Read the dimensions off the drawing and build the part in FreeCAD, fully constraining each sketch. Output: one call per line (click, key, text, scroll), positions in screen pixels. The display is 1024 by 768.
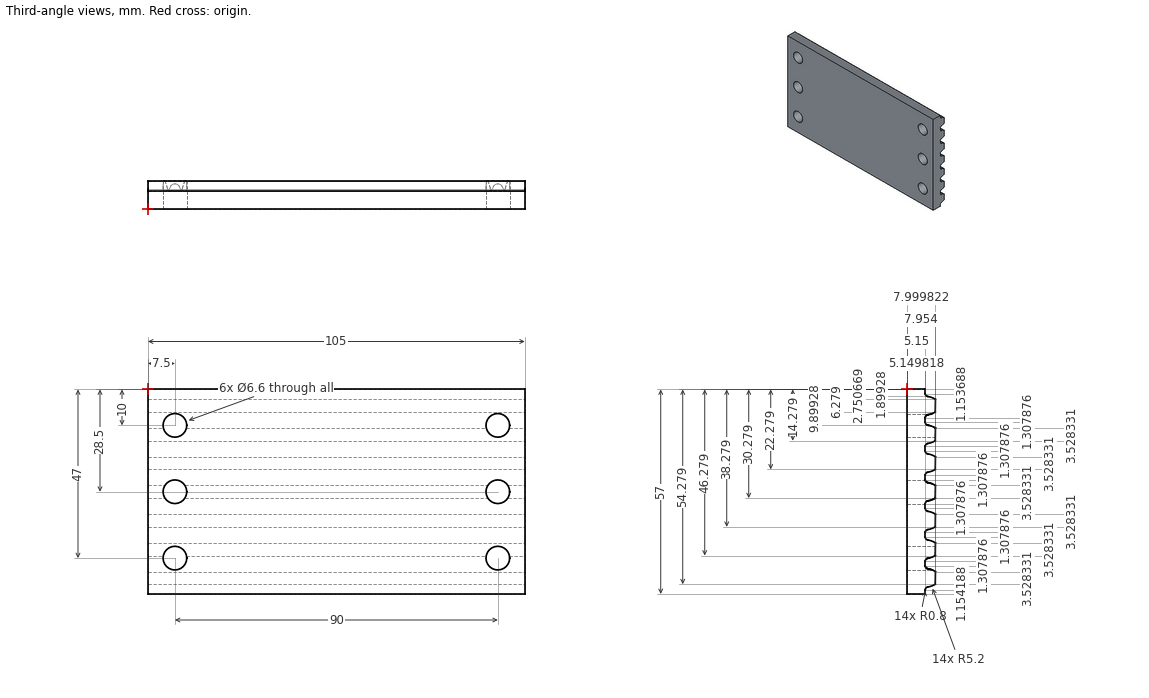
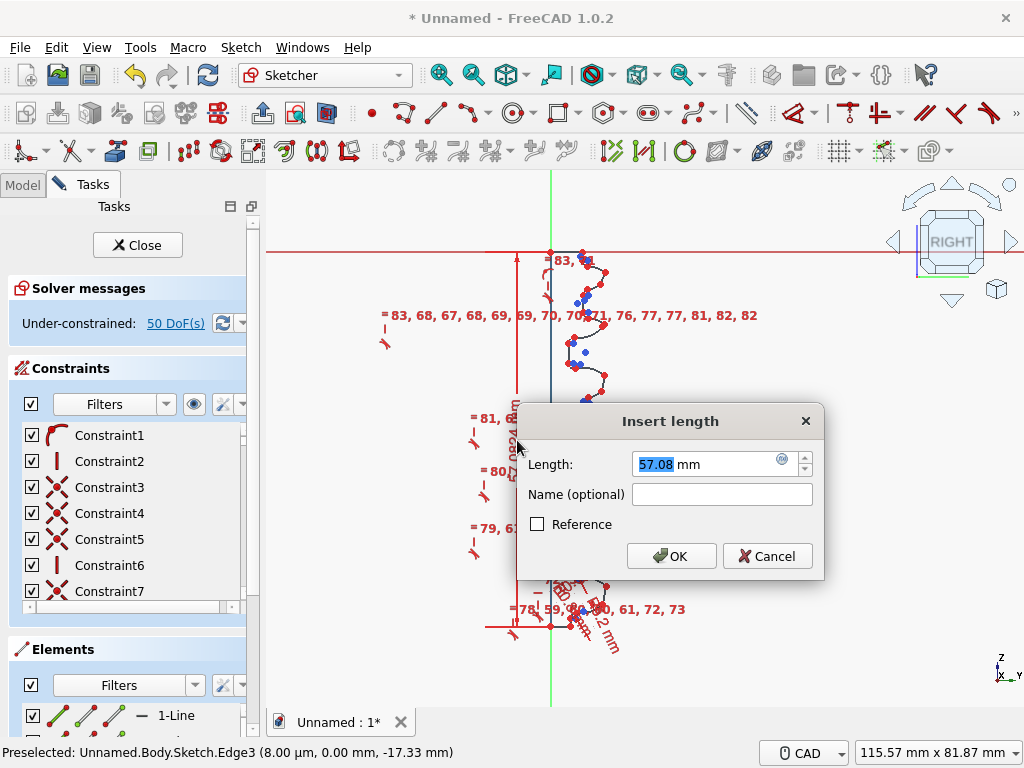
text(57)
key(Return)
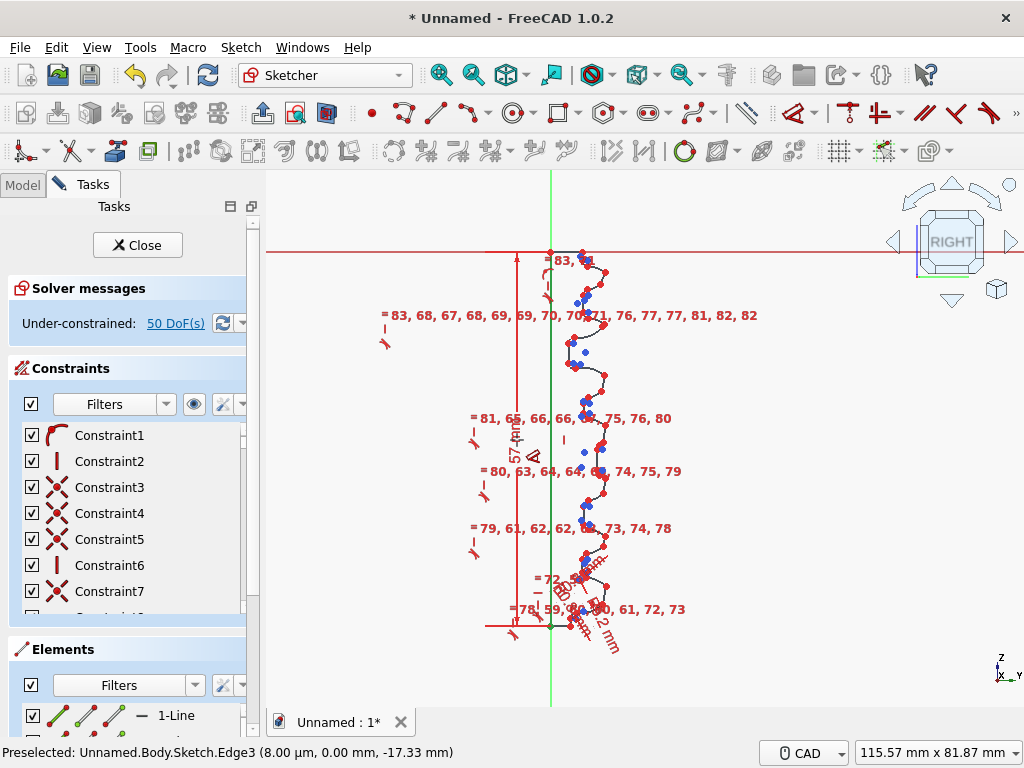
scroll(573, 252, up, 2)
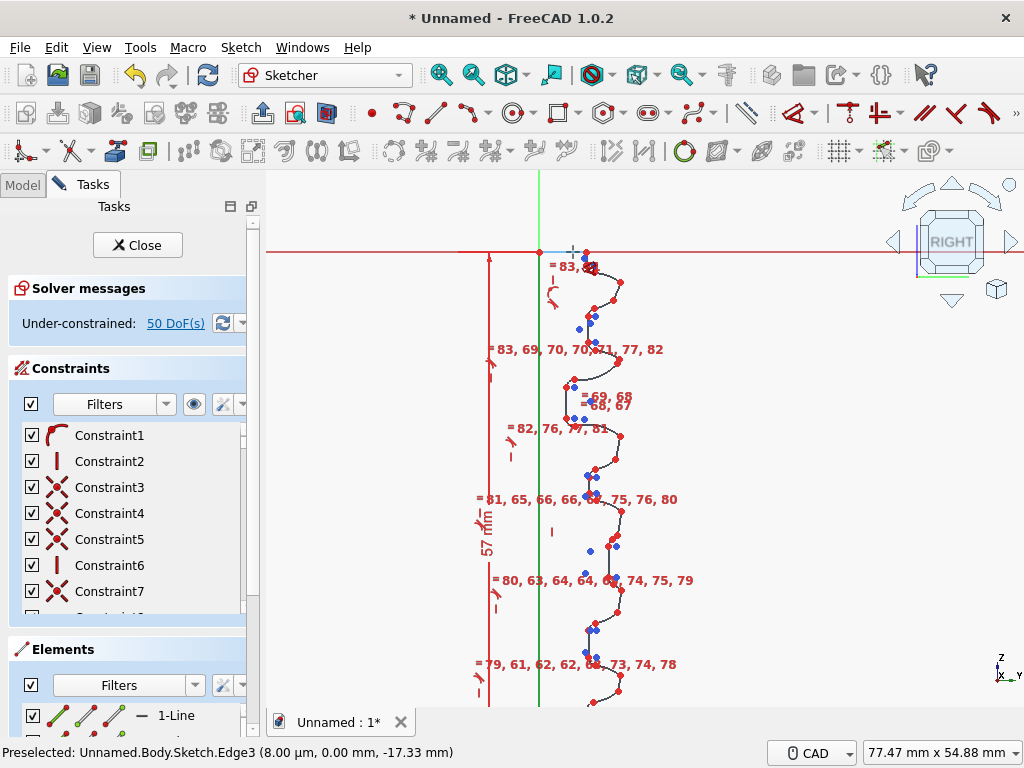
click(573, 252)
click(563, 218)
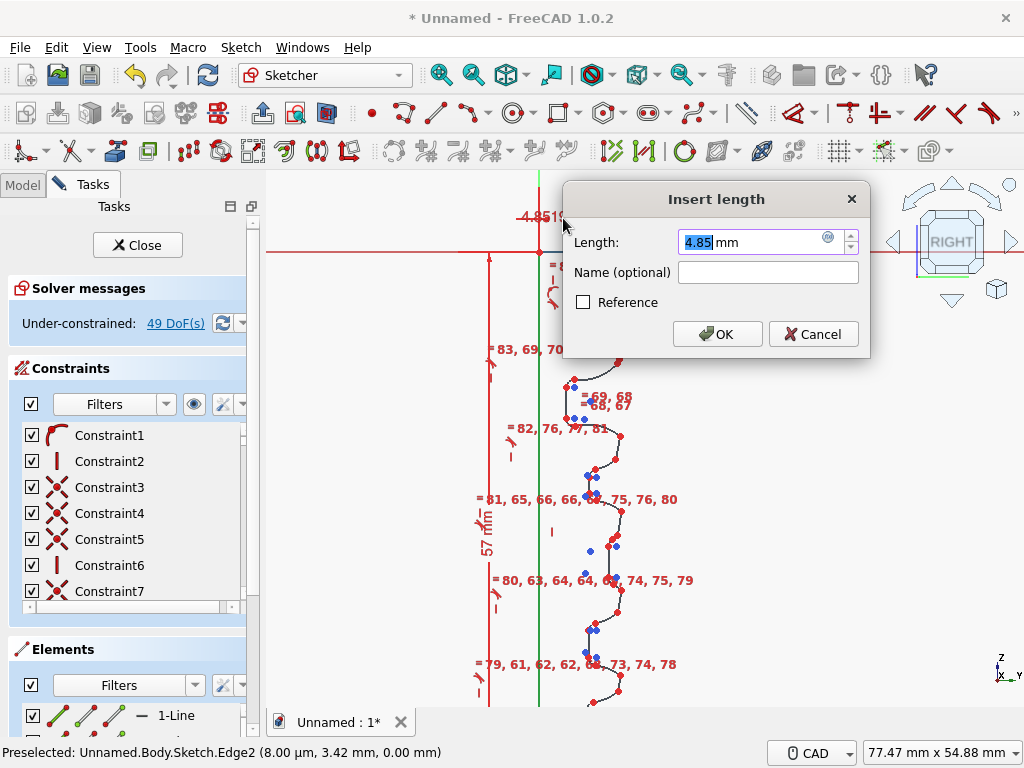
text(5.15)
key(Return)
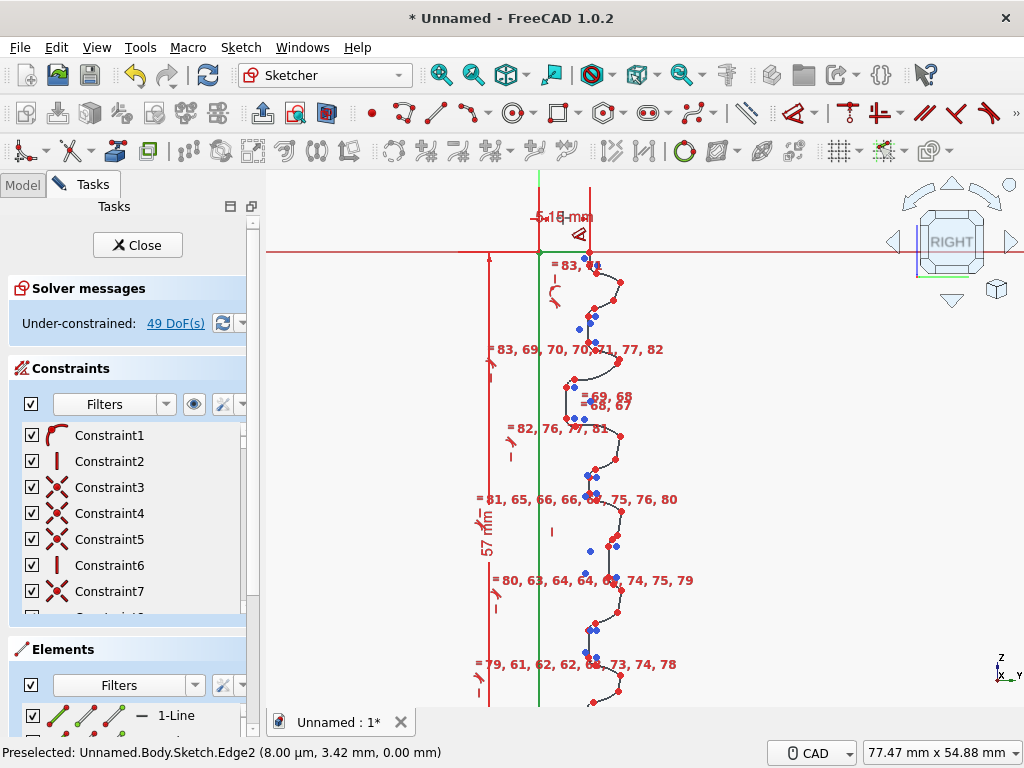
scroll(572, 250, down, 2)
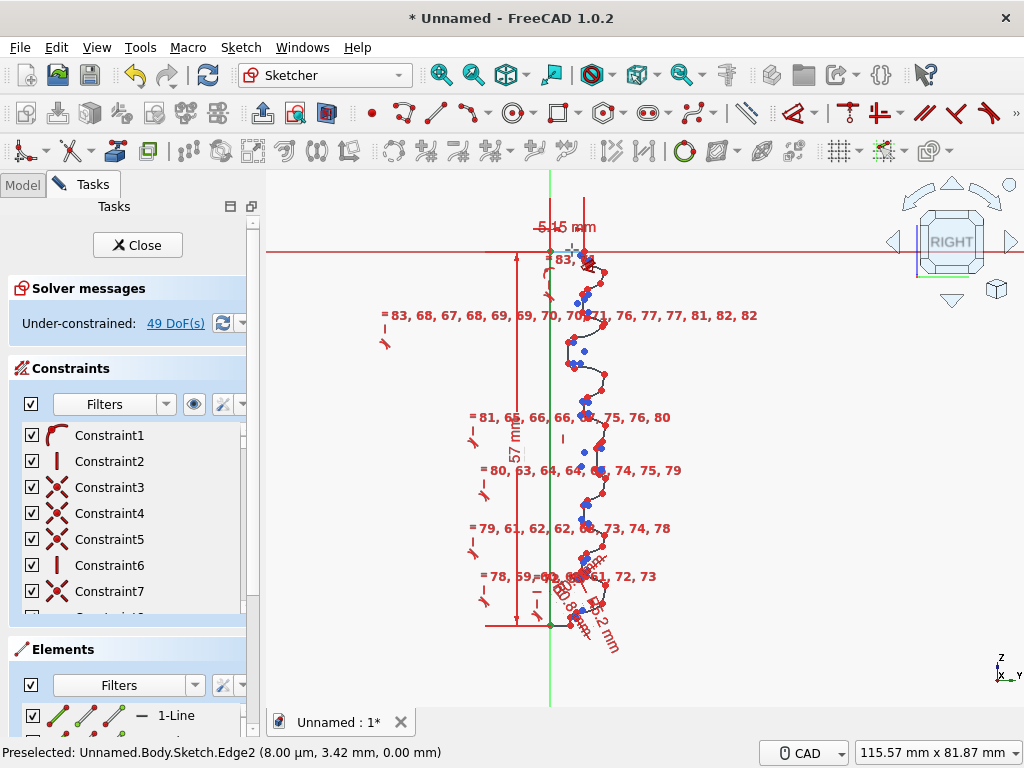
scroll(558, 626, up, 3)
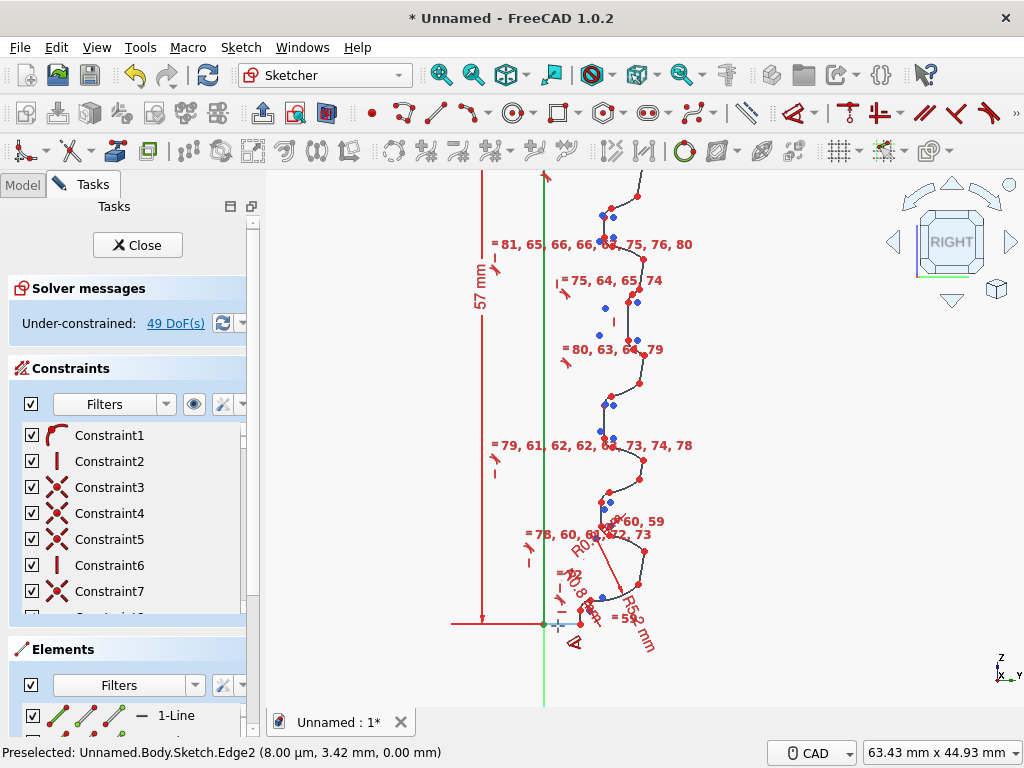
click(558, 624)
click(562, 658)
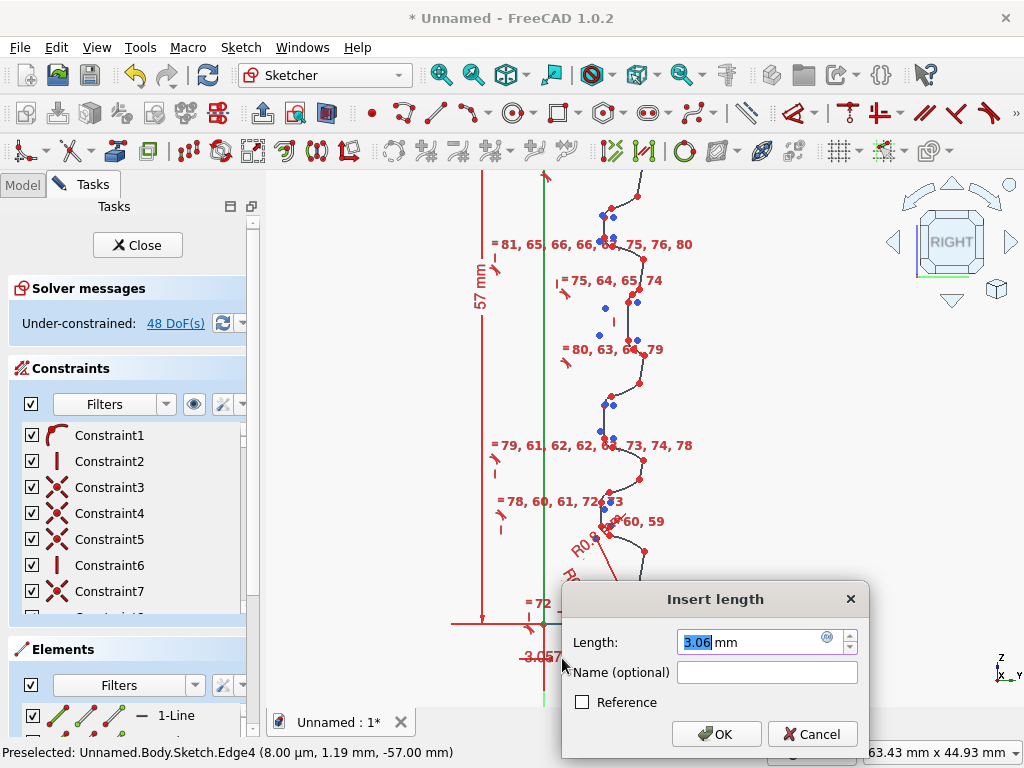
text(5.15)
key(Return)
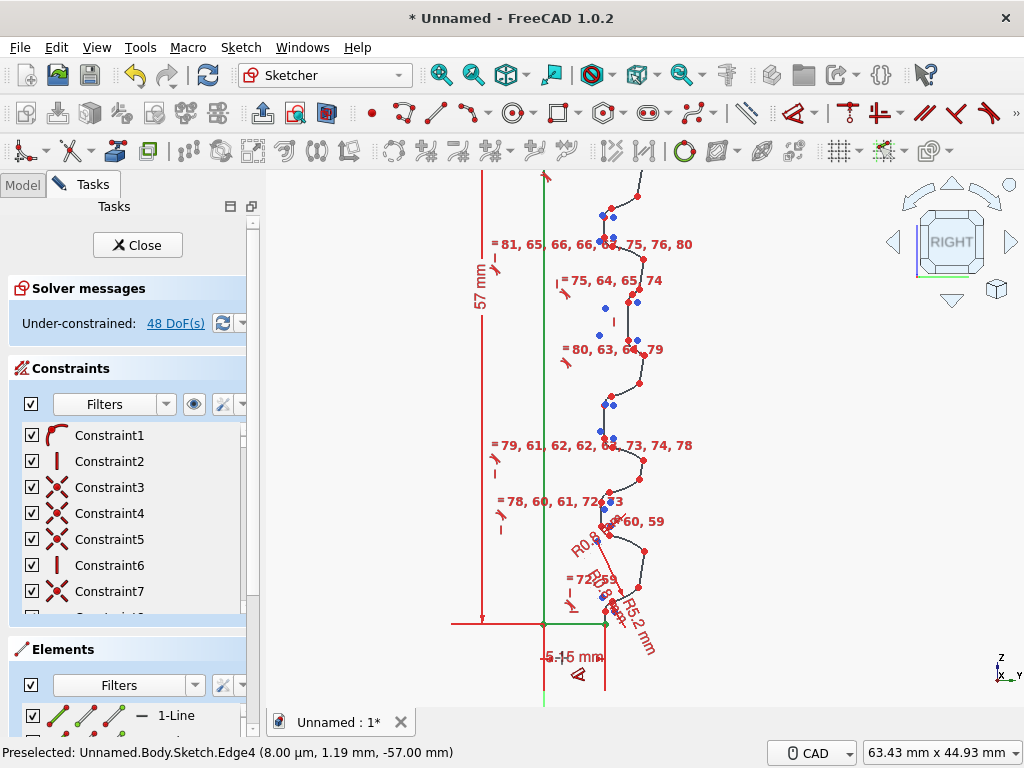
scroll(601, 526, up, 2)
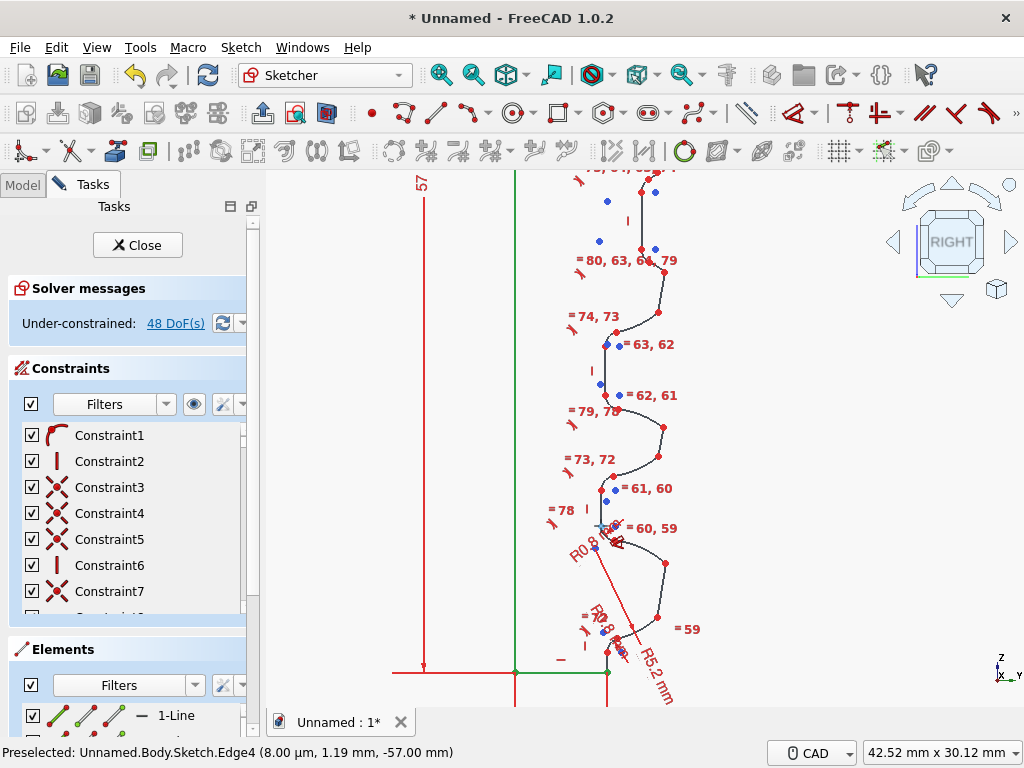
click(601, 526)
click(558, 584)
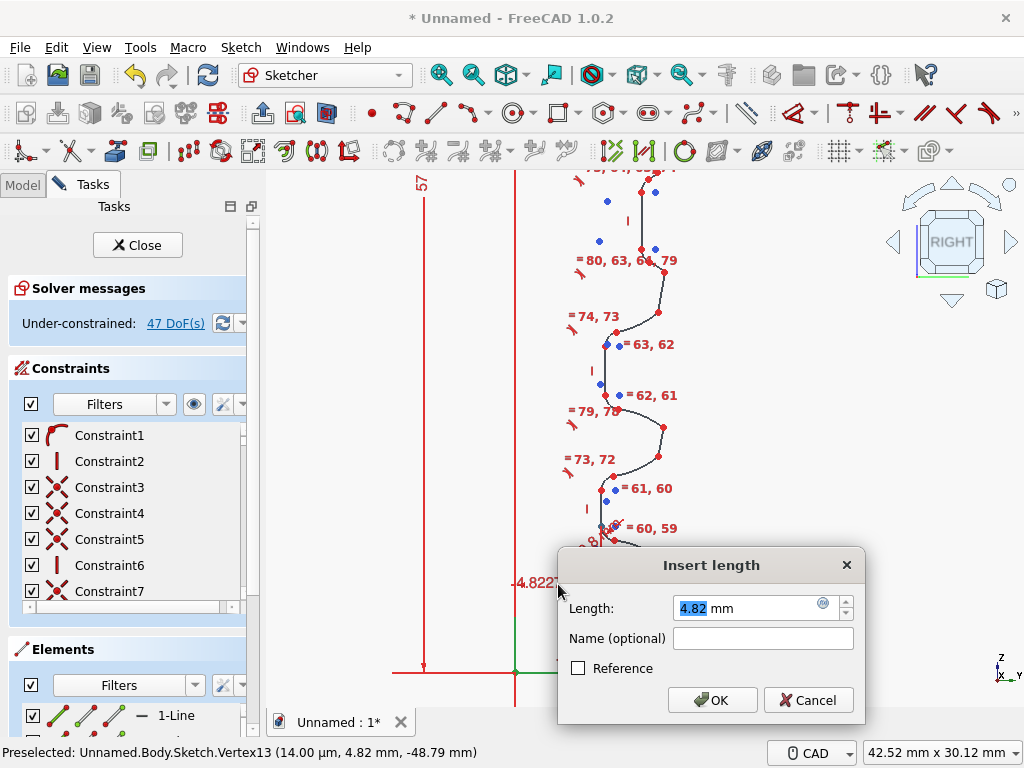
text(5.15)
key(Return)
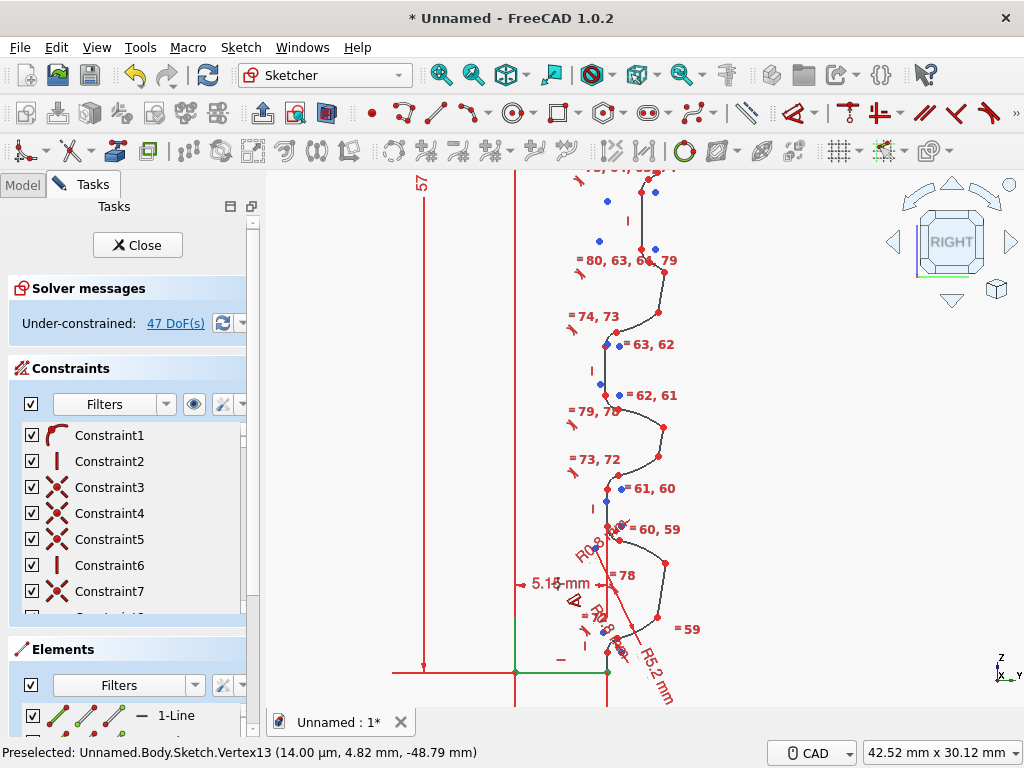
click(605, 395)
click(560, 429)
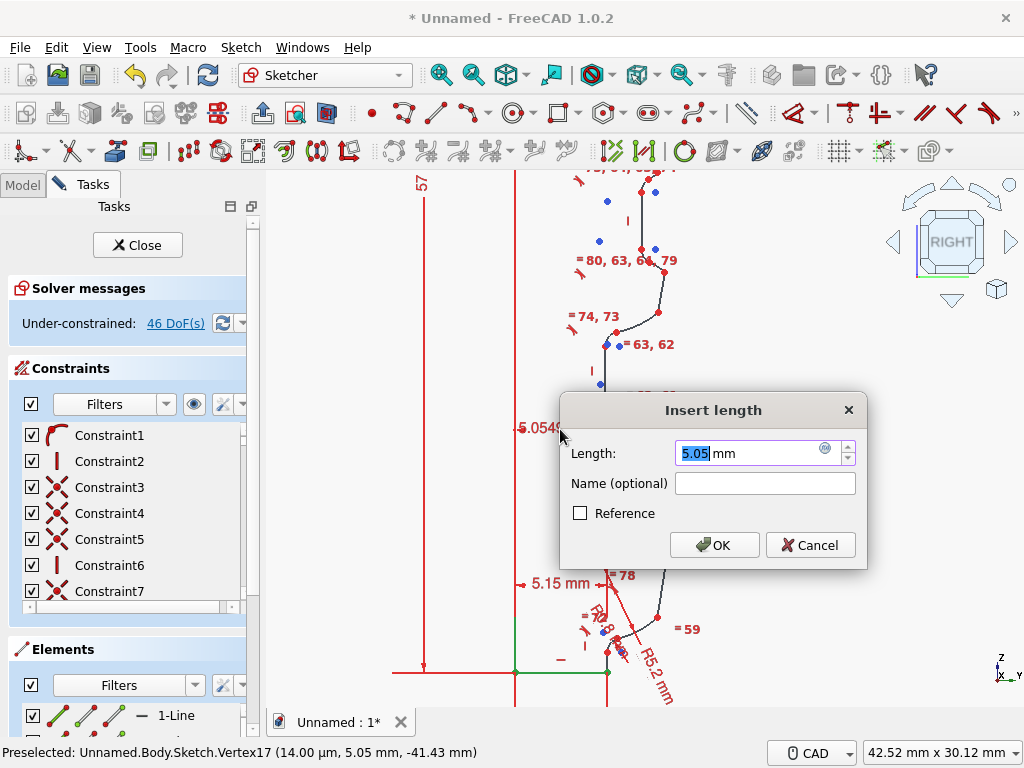
text(5.15)
key(Return)